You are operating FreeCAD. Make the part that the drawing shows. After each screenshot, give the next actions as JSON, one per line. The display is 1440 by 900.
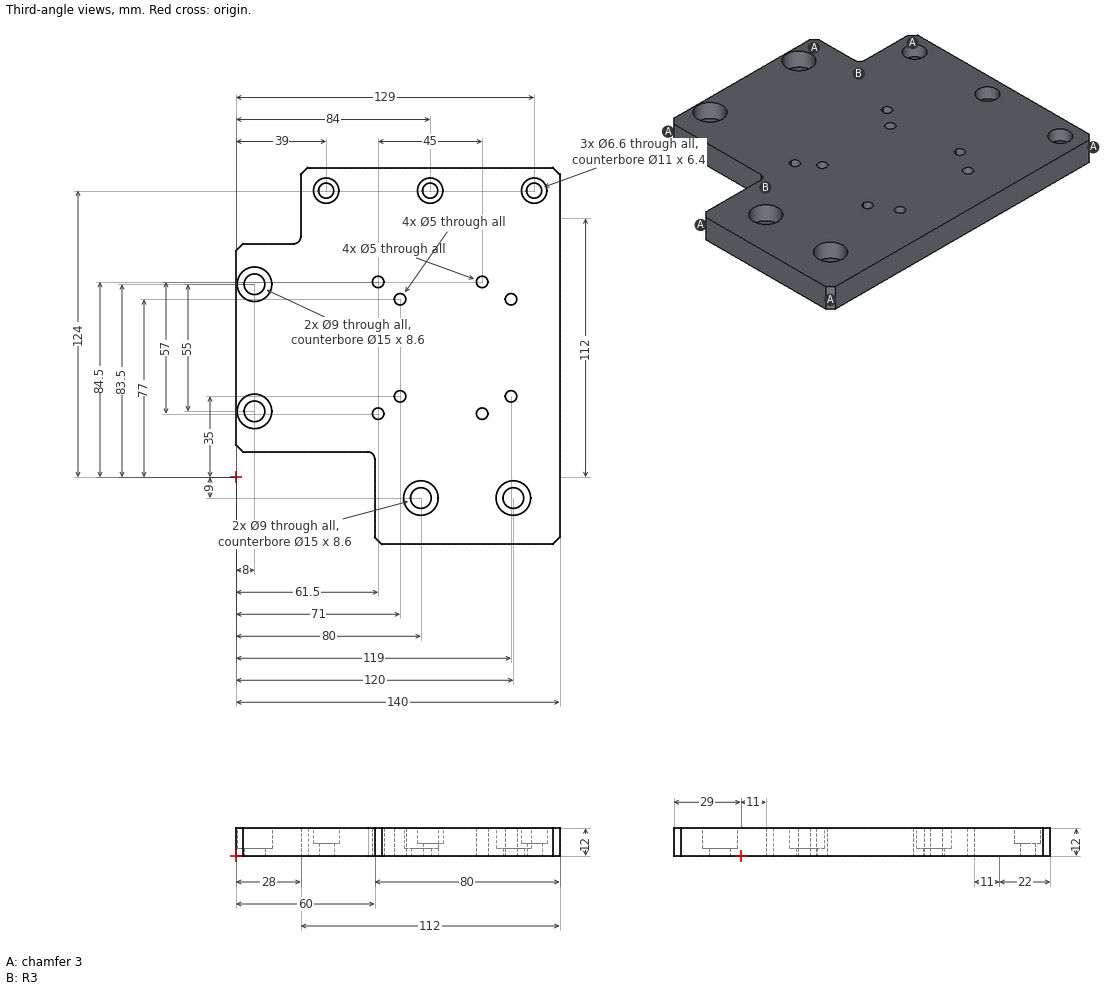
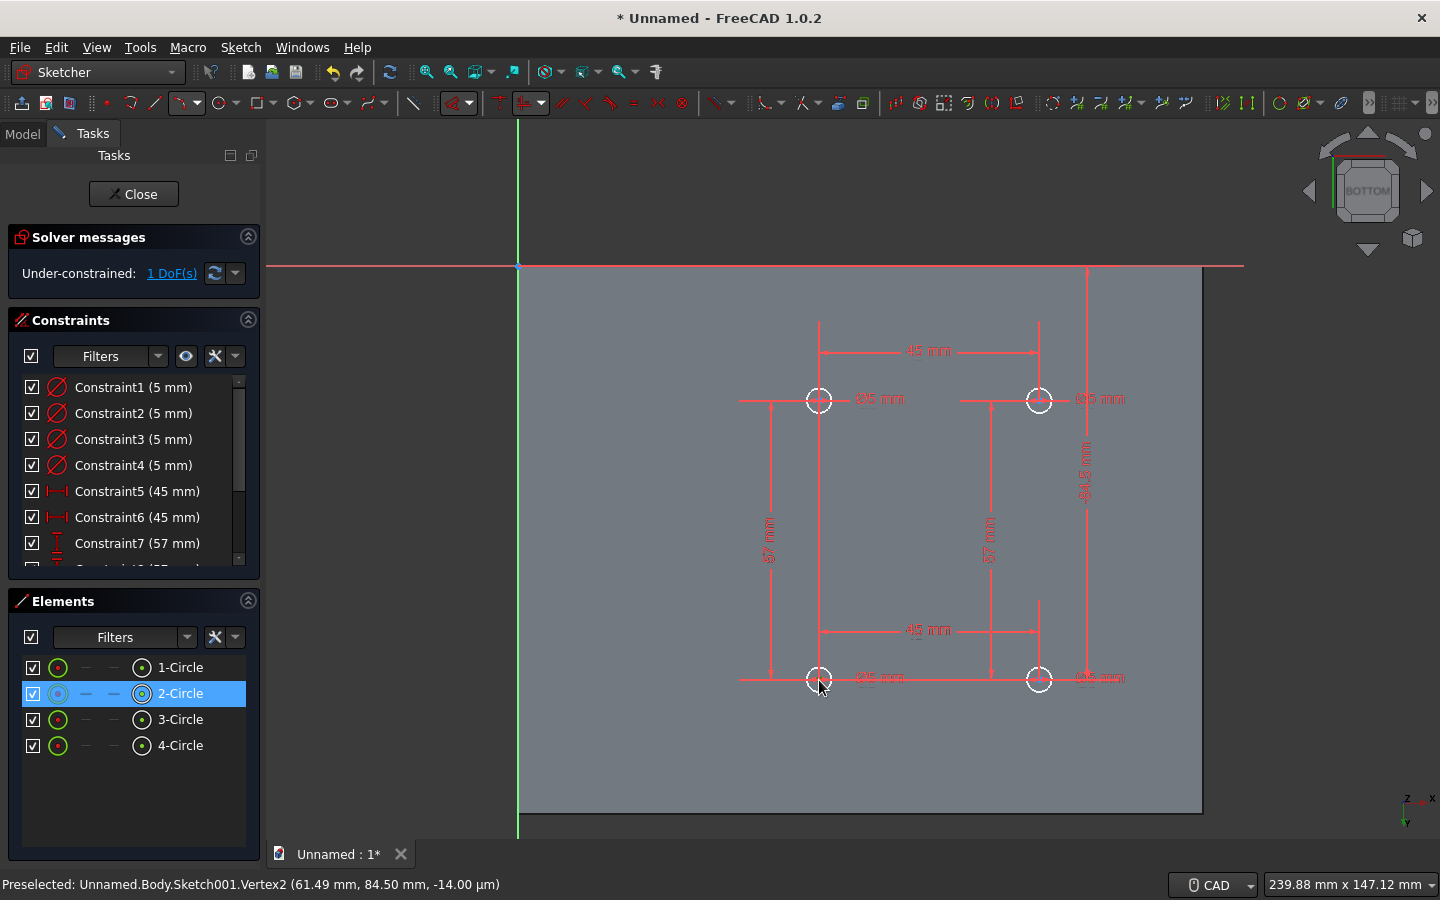
{"action": "left_click", "coordinate": [472, 104]}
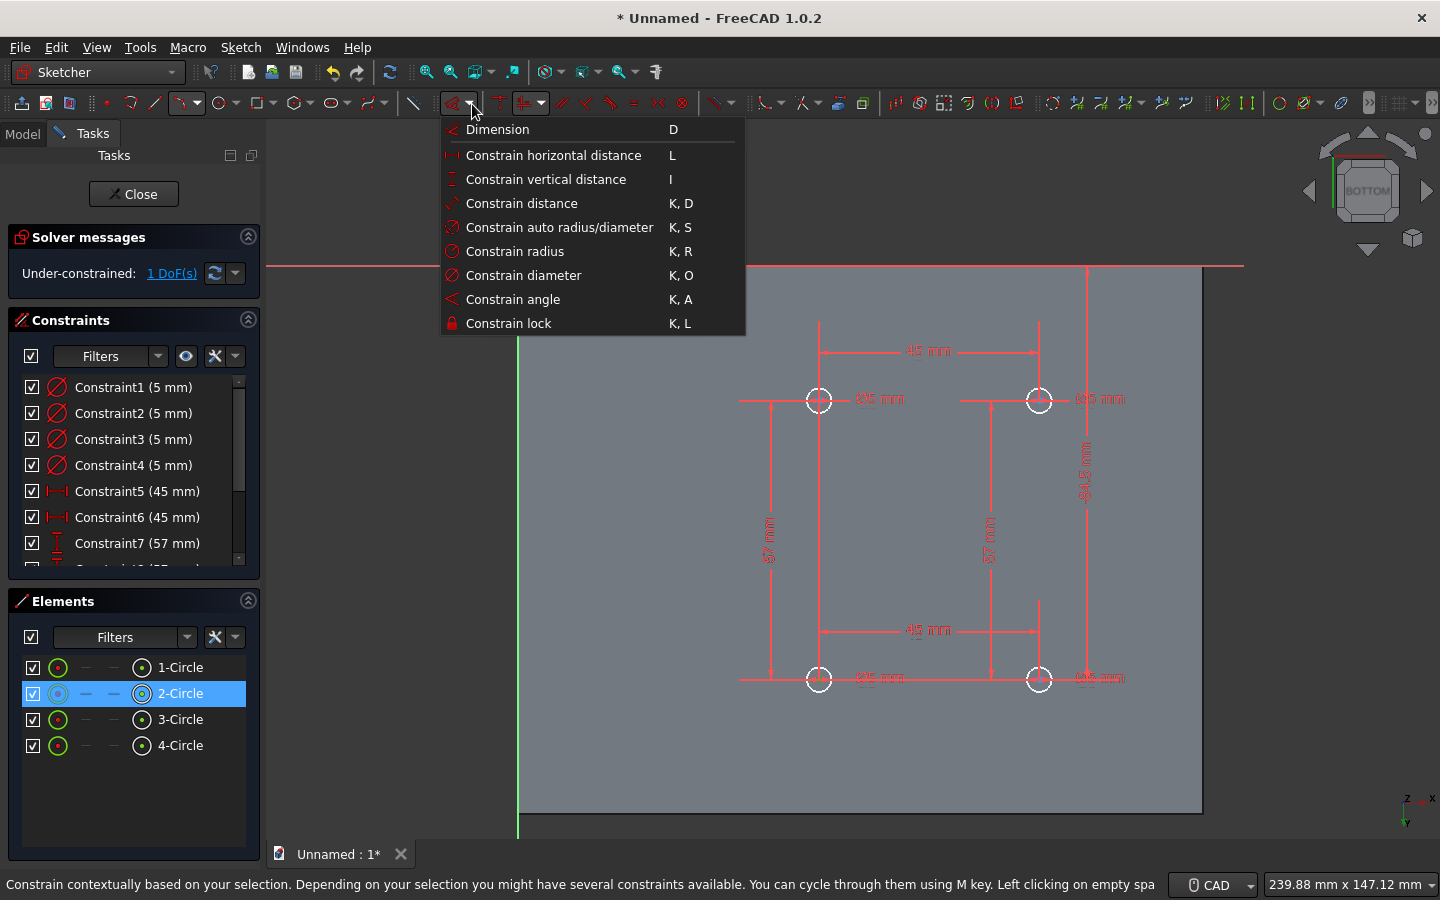
{"action": "left_click", "coordinate": [593, 155]}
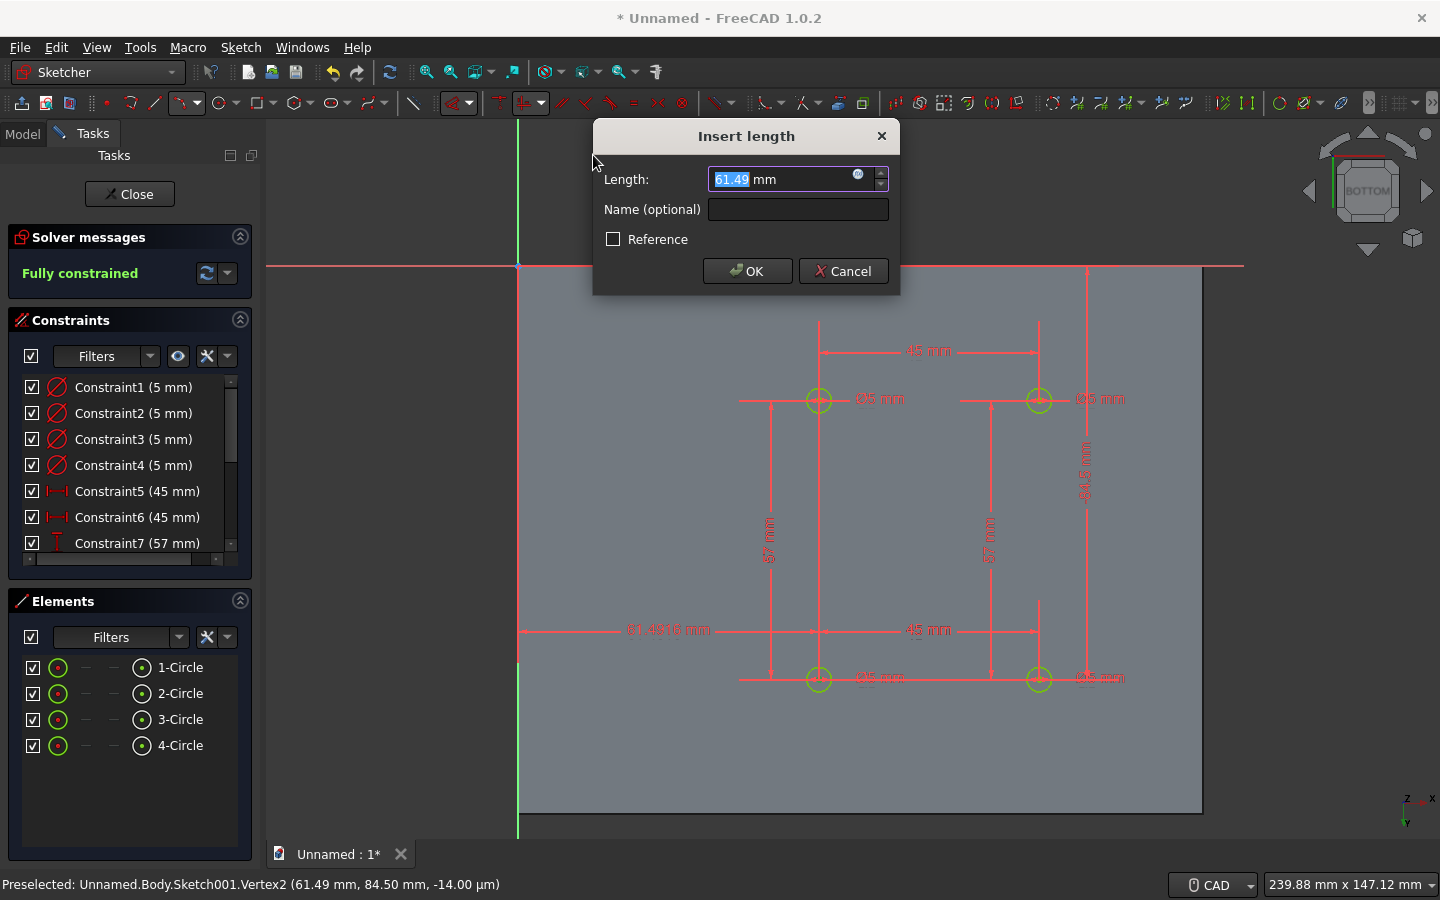
{"action": "type", "text": "61.5"}
{"action": "key", "text": "Return"}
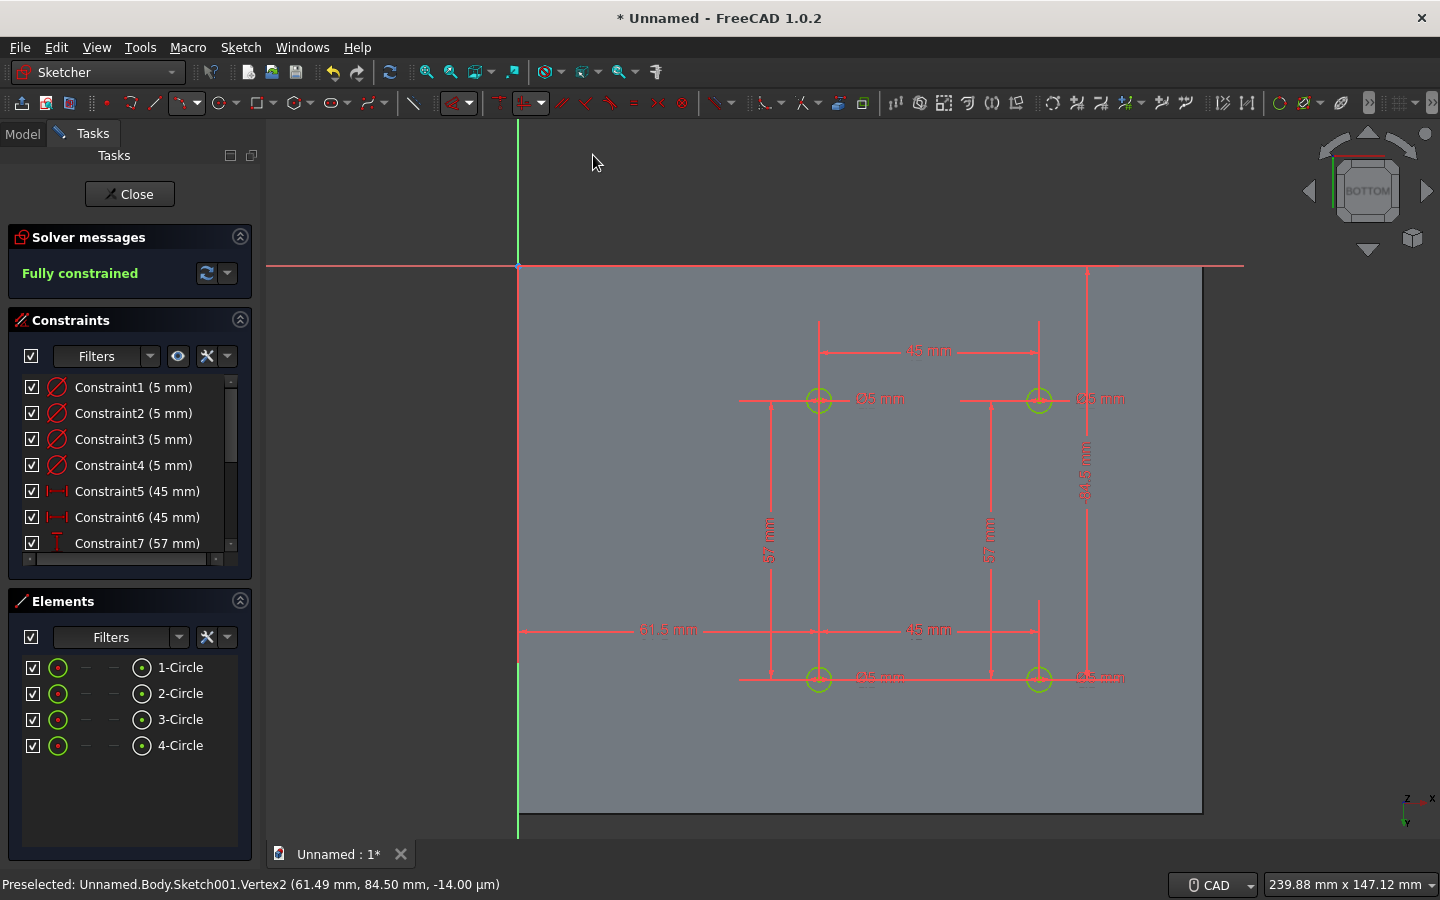
{"action": "left_click", "coordinate": [130, 194]}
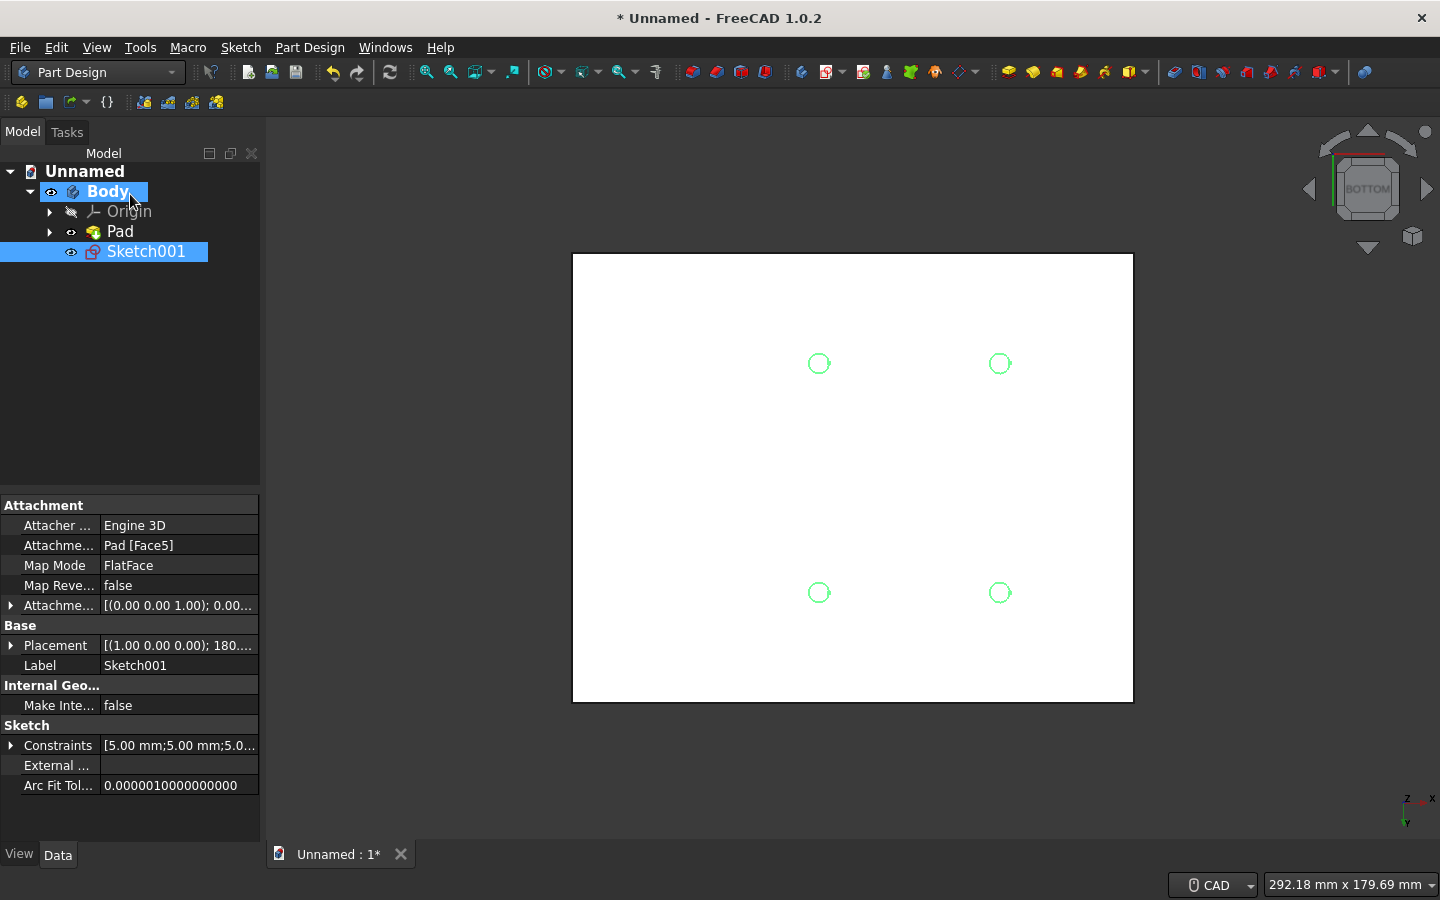
{"action": "left_click", "coordinate": [1200, 72]}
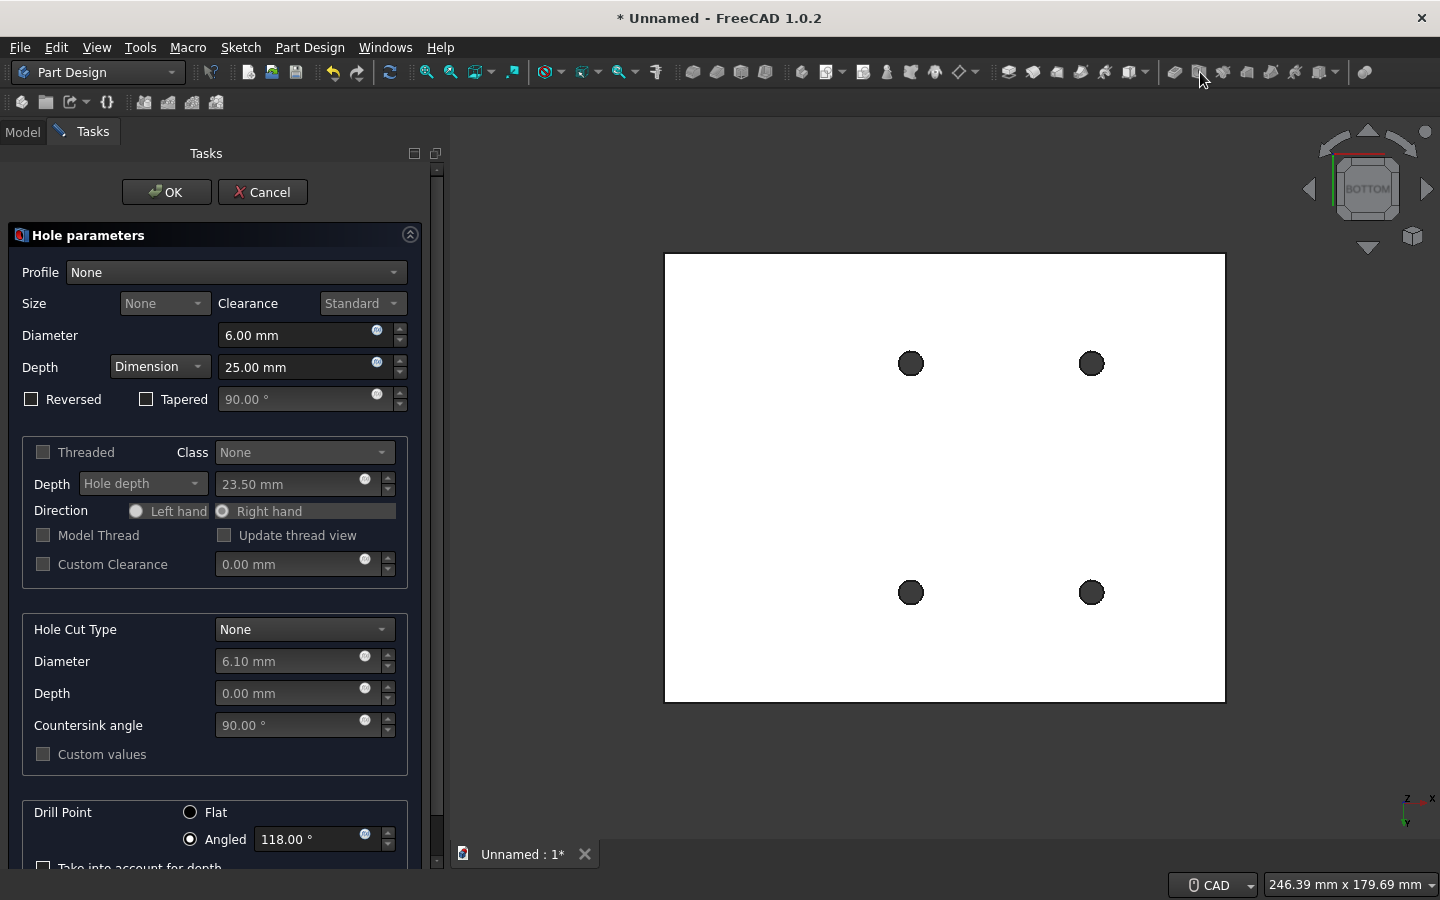
{"action": "triple_click", "coordinate": [305, 335]}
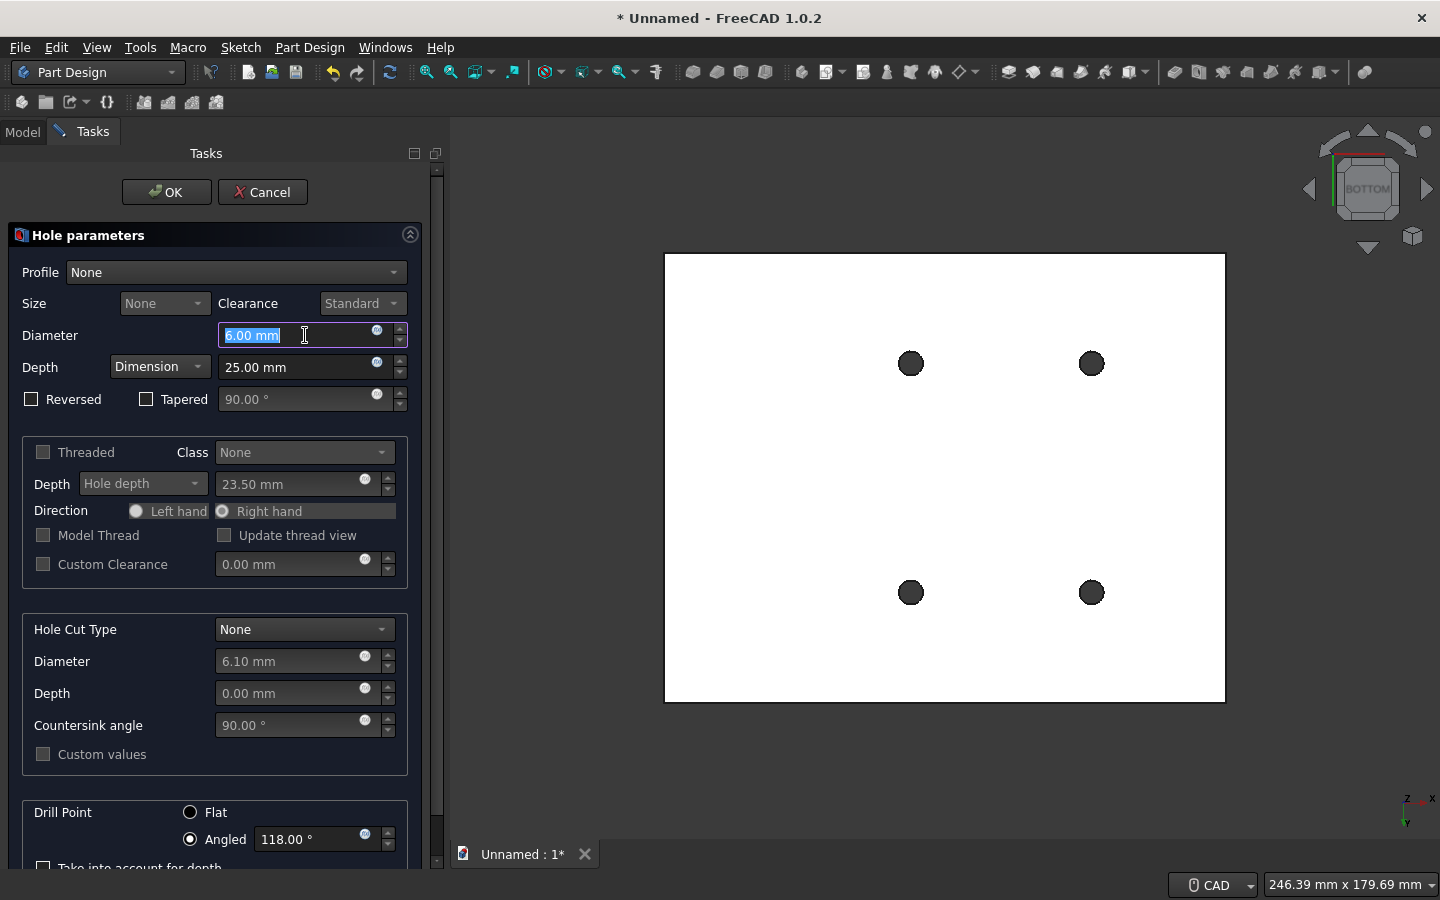
{"action": "type", "text": "5"}
{"action": "key", "text": "Tab"}